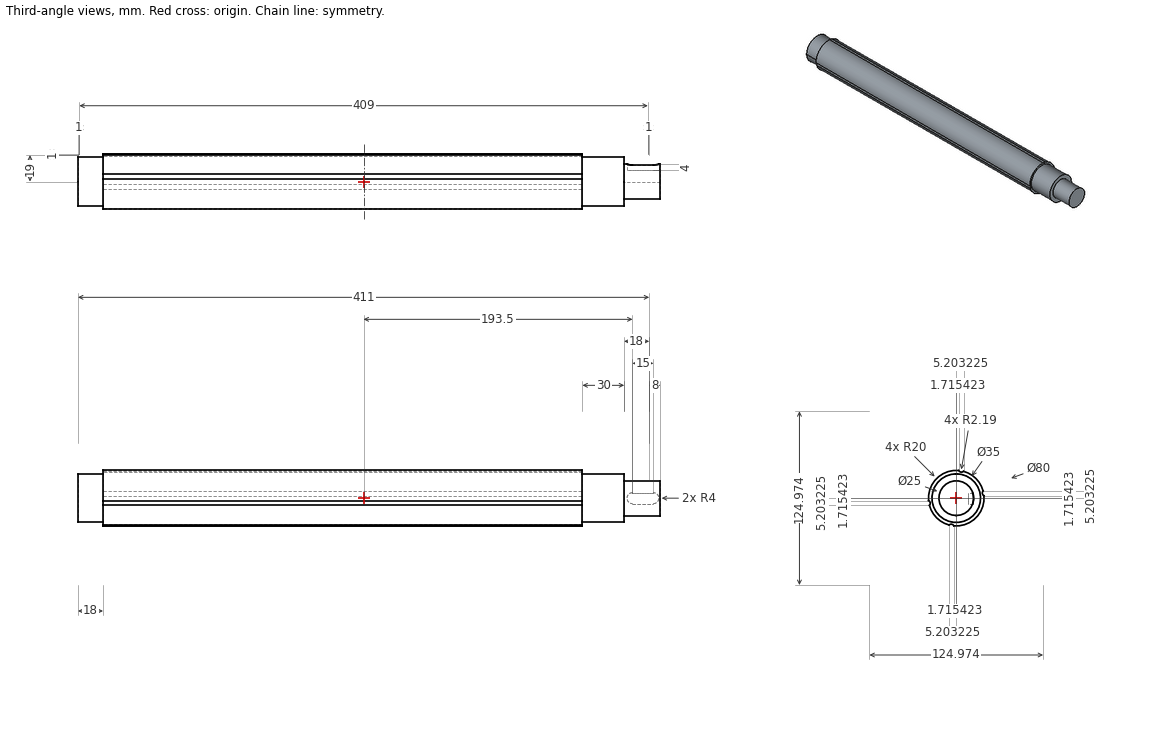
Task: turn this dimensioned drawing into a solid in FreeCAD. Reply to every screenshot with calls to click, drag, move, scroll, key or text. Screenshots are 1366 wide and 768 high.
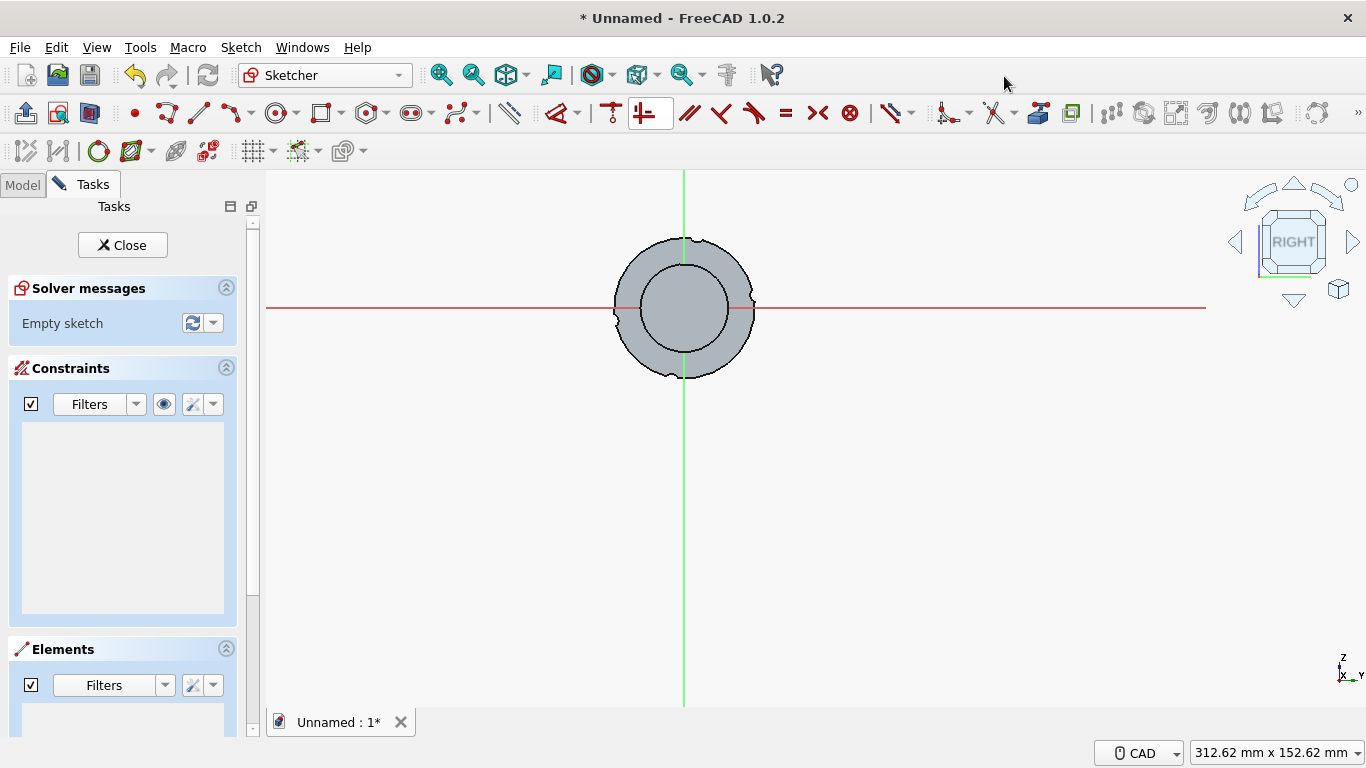
scroll(876, 679, down, 2)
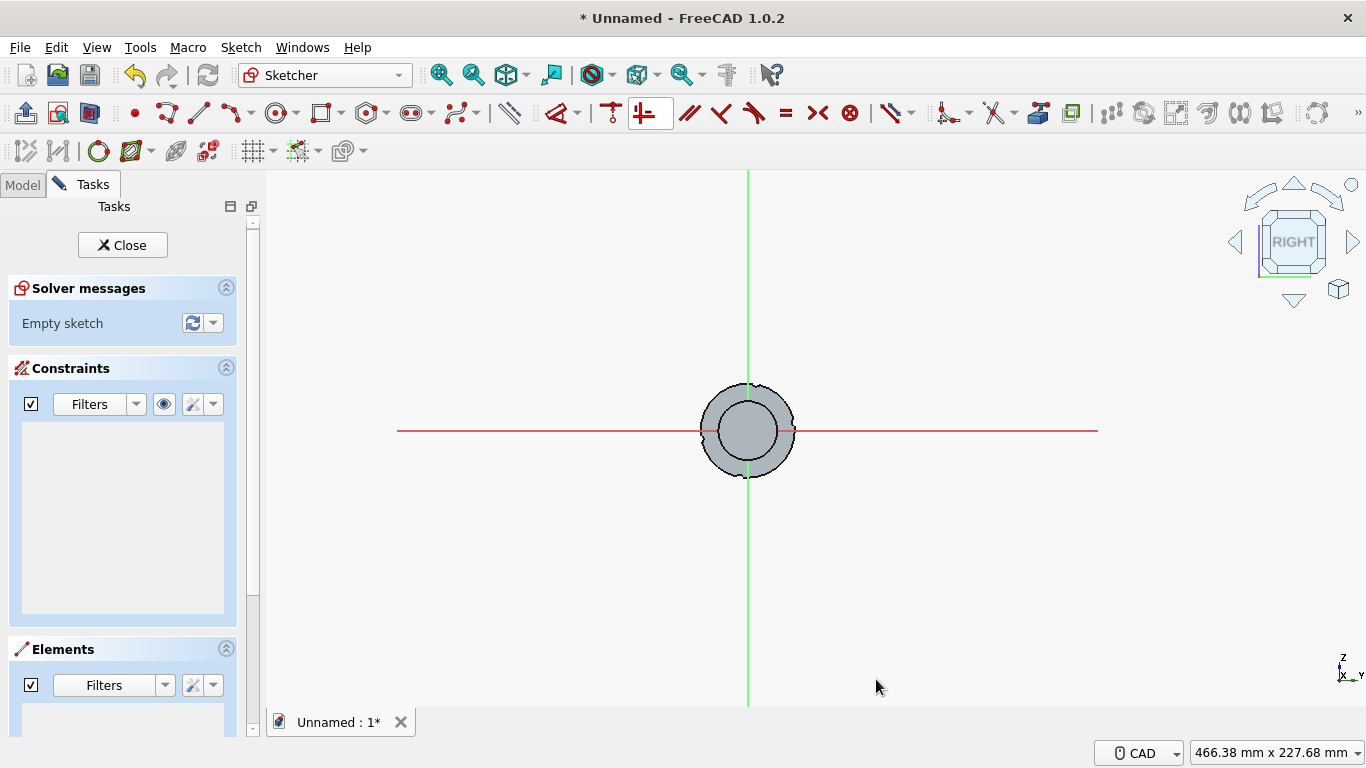
key(g)
key(v)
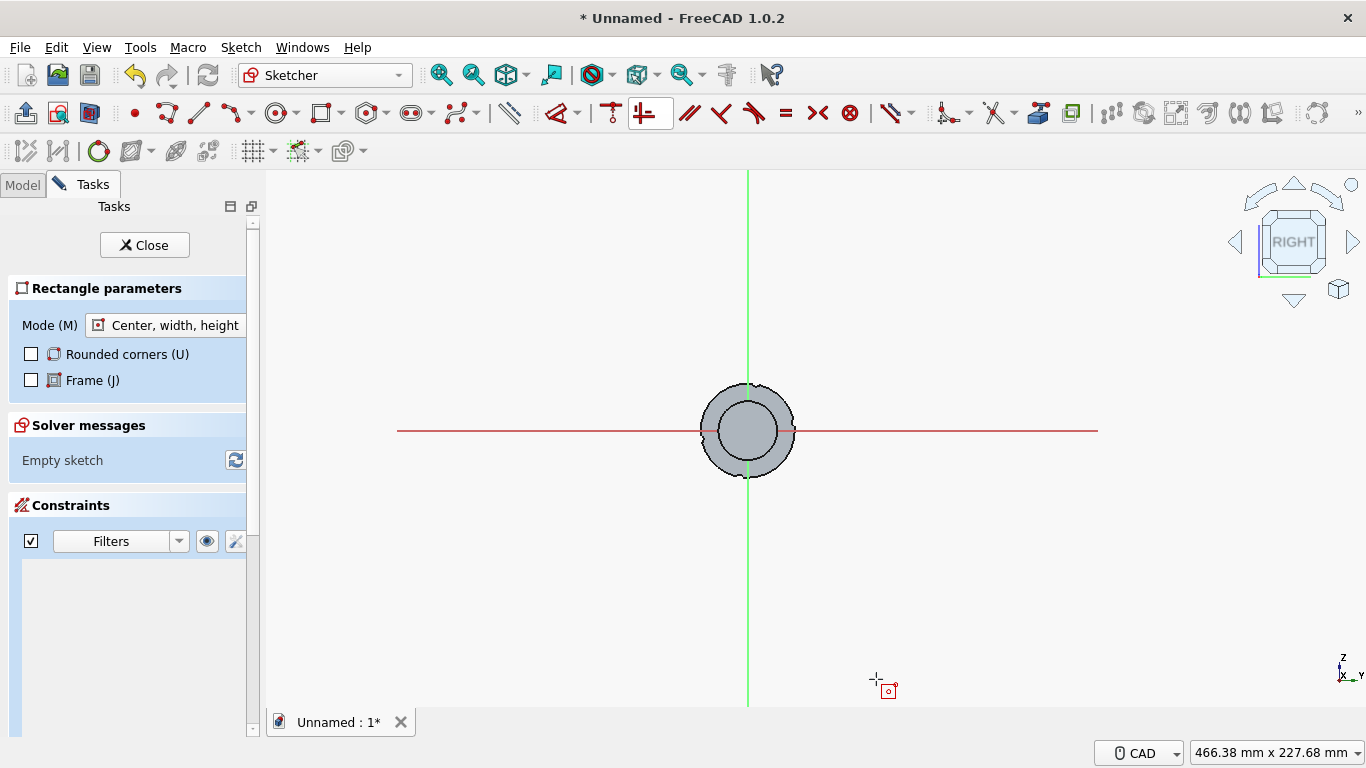
click(748, 431)
click(895, 283)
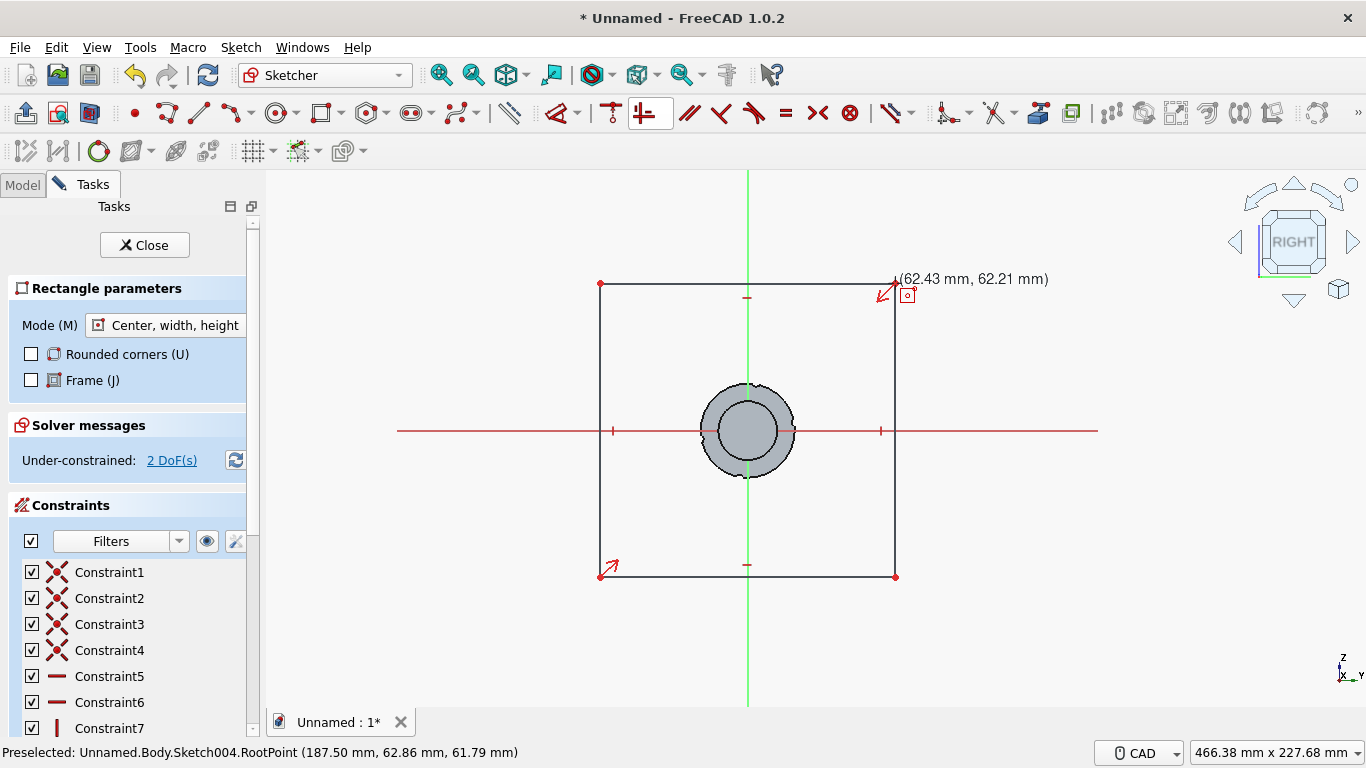
click(276, 114)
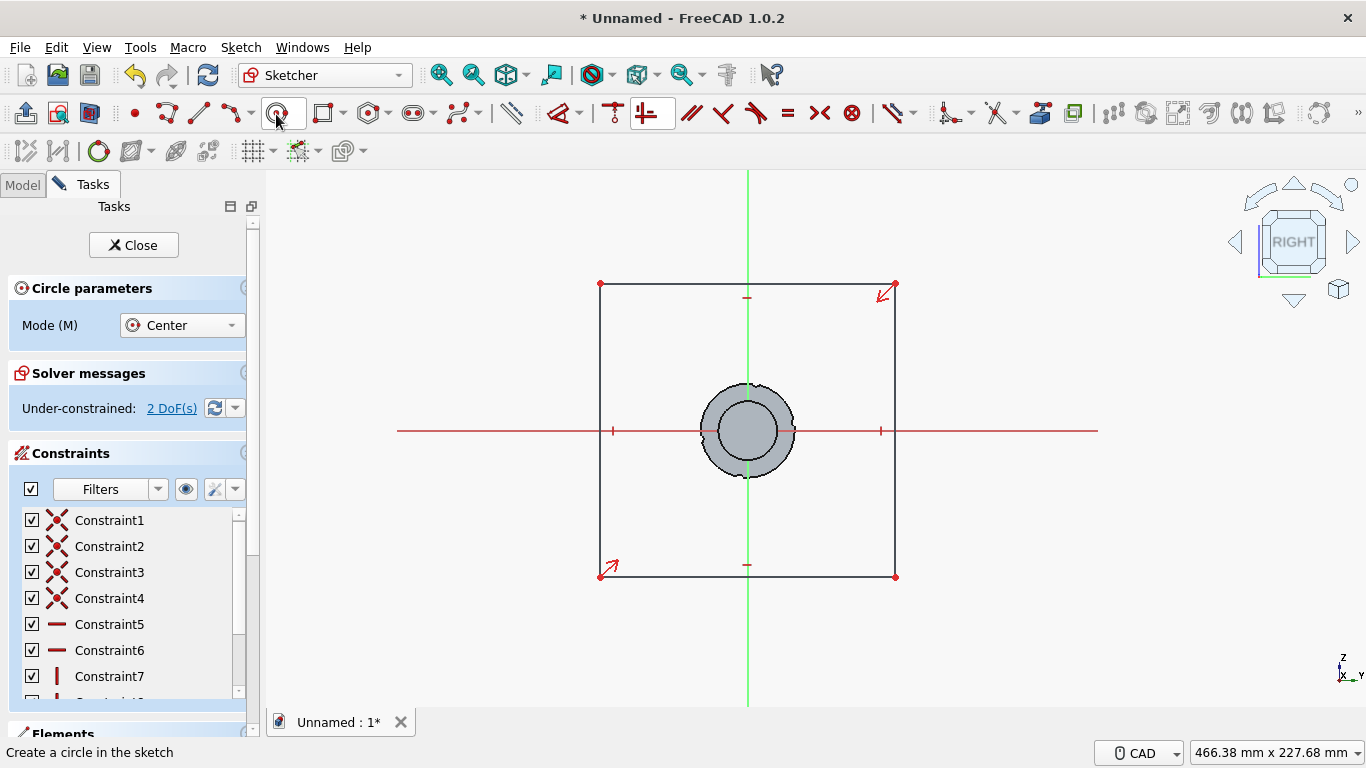
click(748, 431)
click(777, 402)
key(Escape)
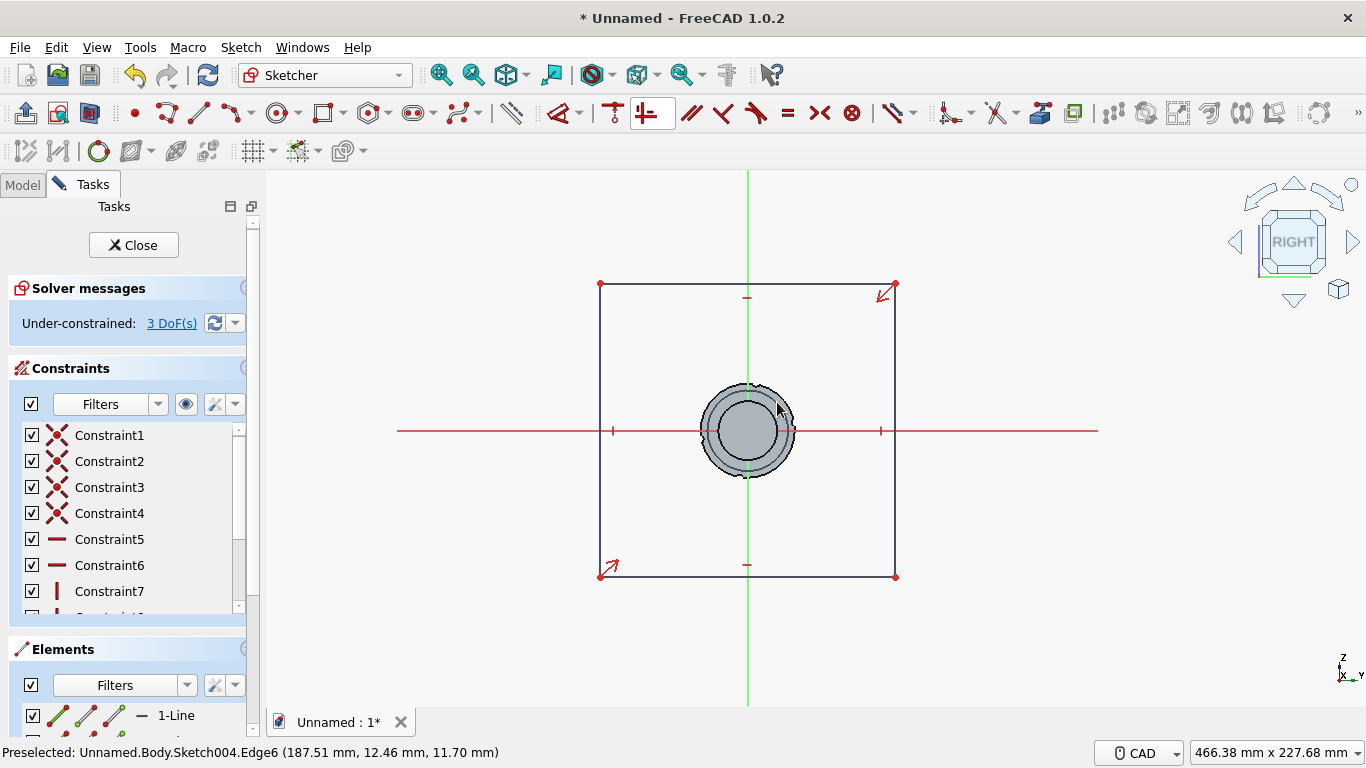
key(d)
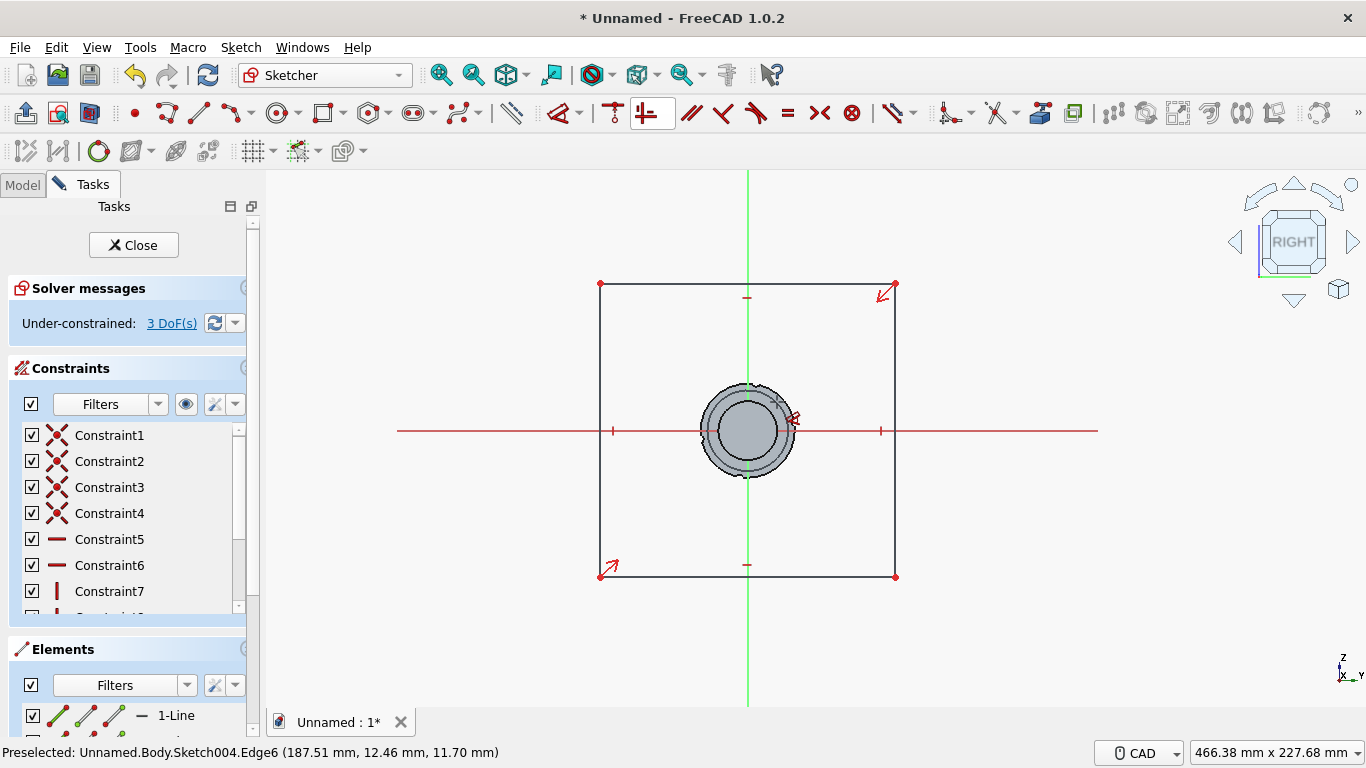
click(776, 402)
click(798, 379)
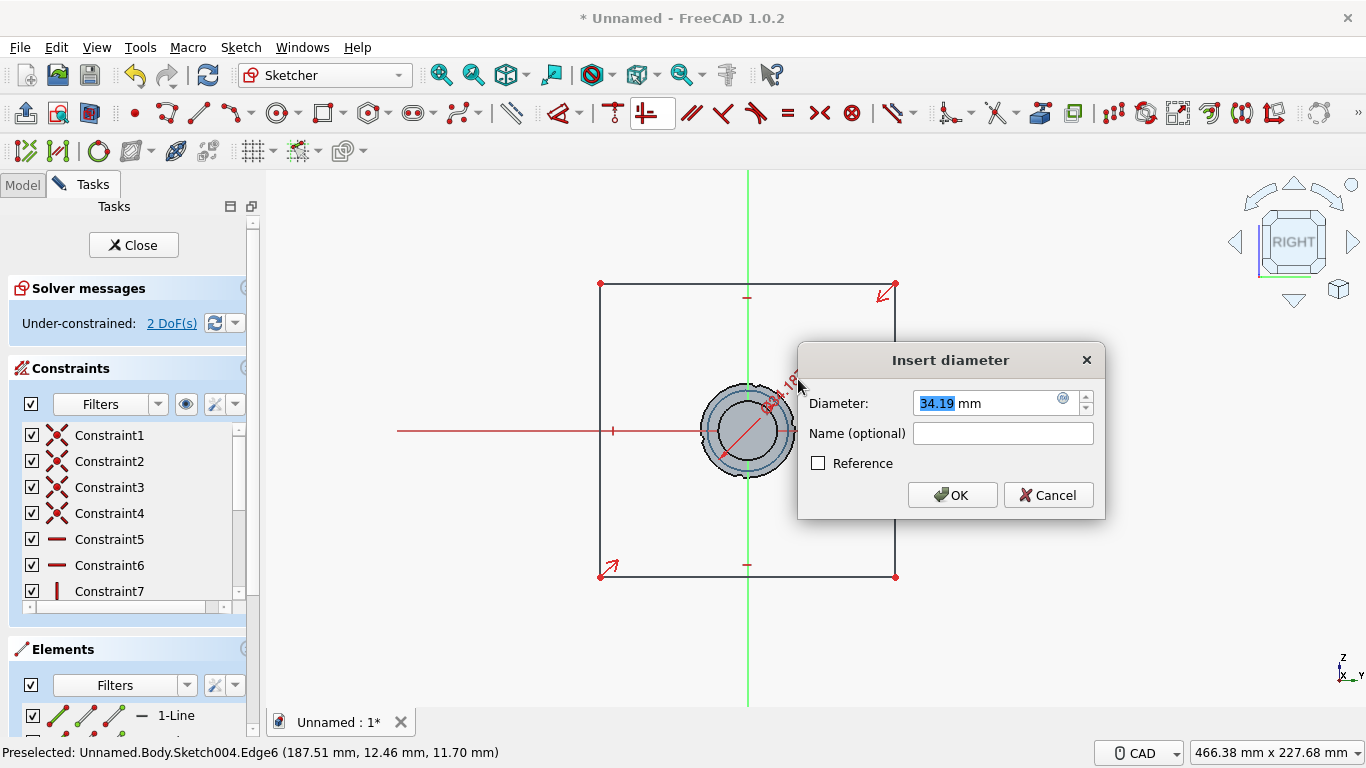
text(35)
key(Return)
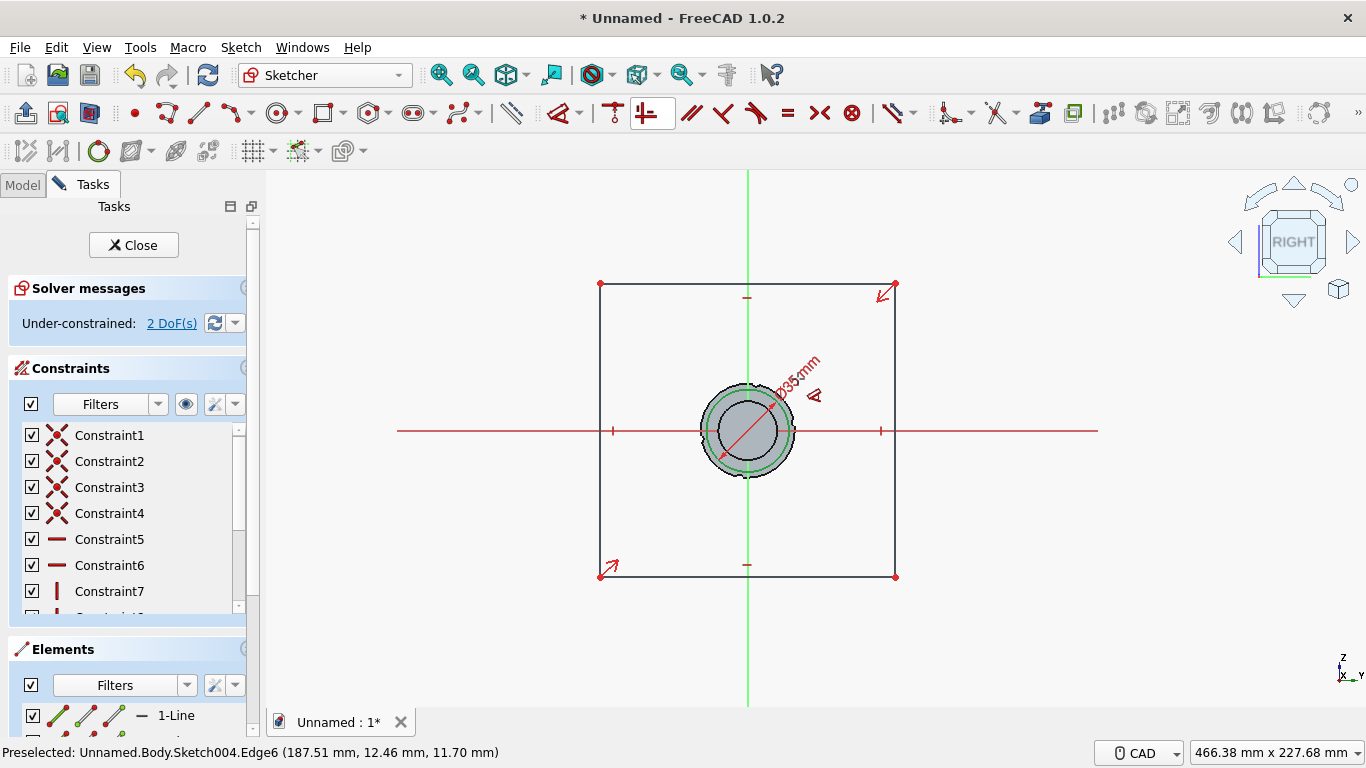
click(689, 577)
click(680, 611)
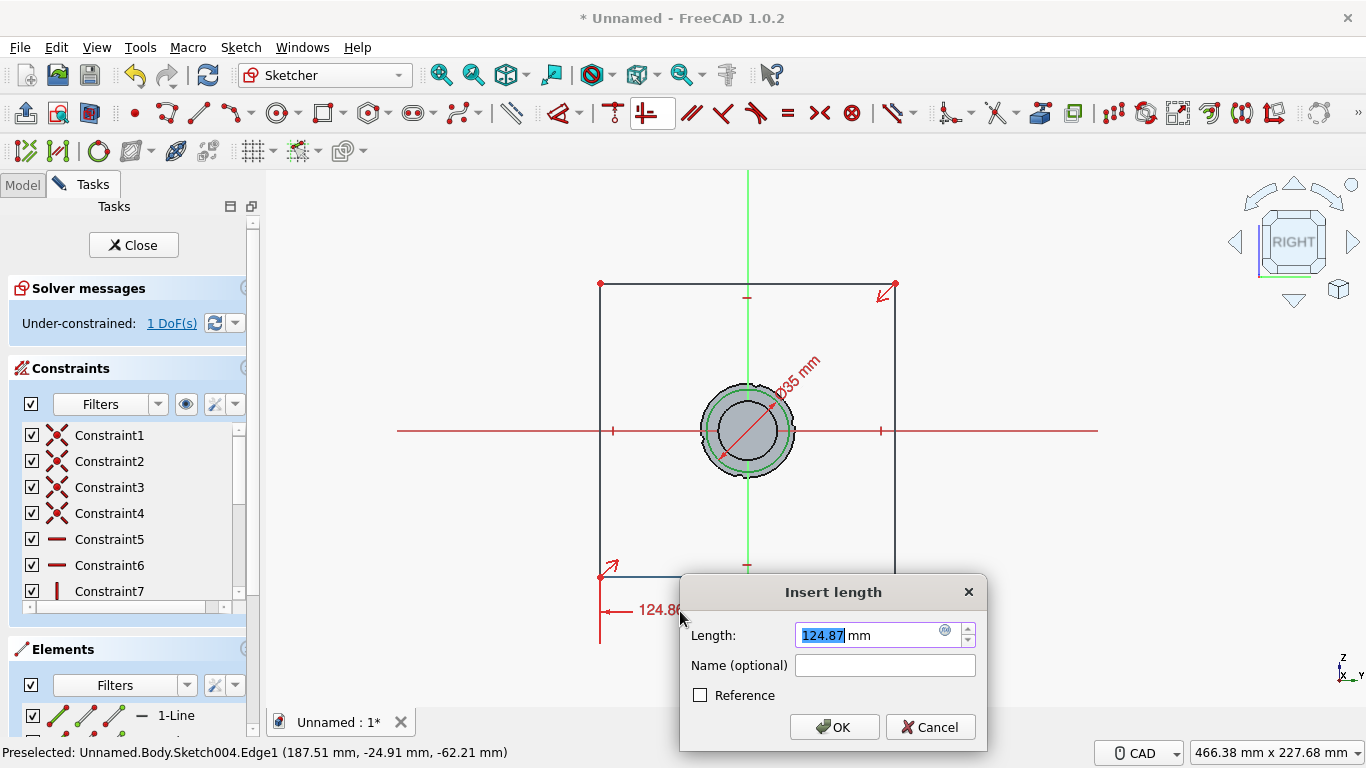
text(124.974)
key(Return)